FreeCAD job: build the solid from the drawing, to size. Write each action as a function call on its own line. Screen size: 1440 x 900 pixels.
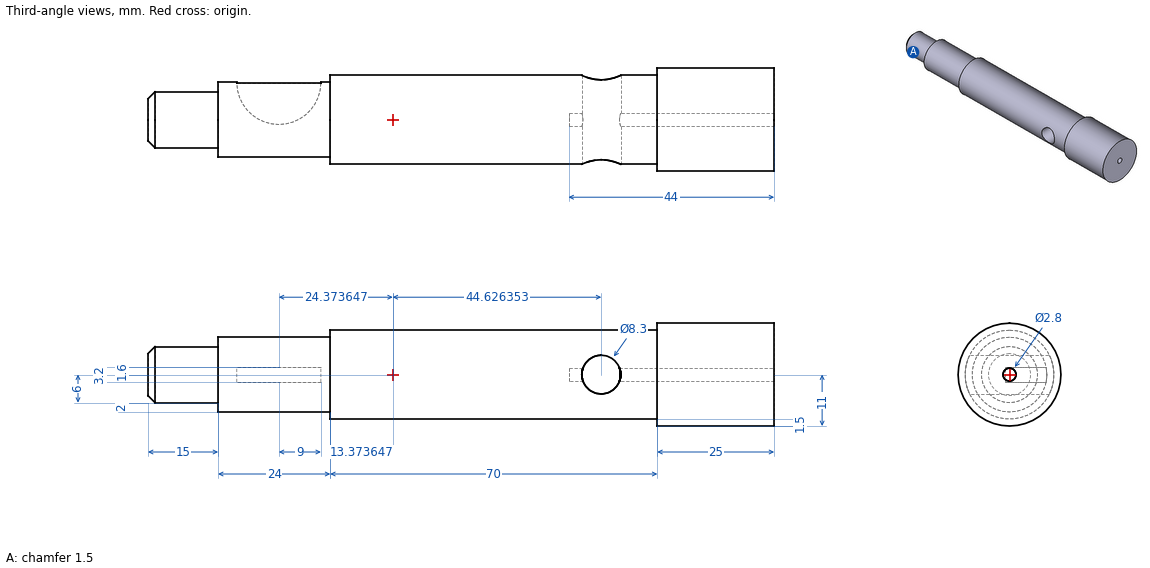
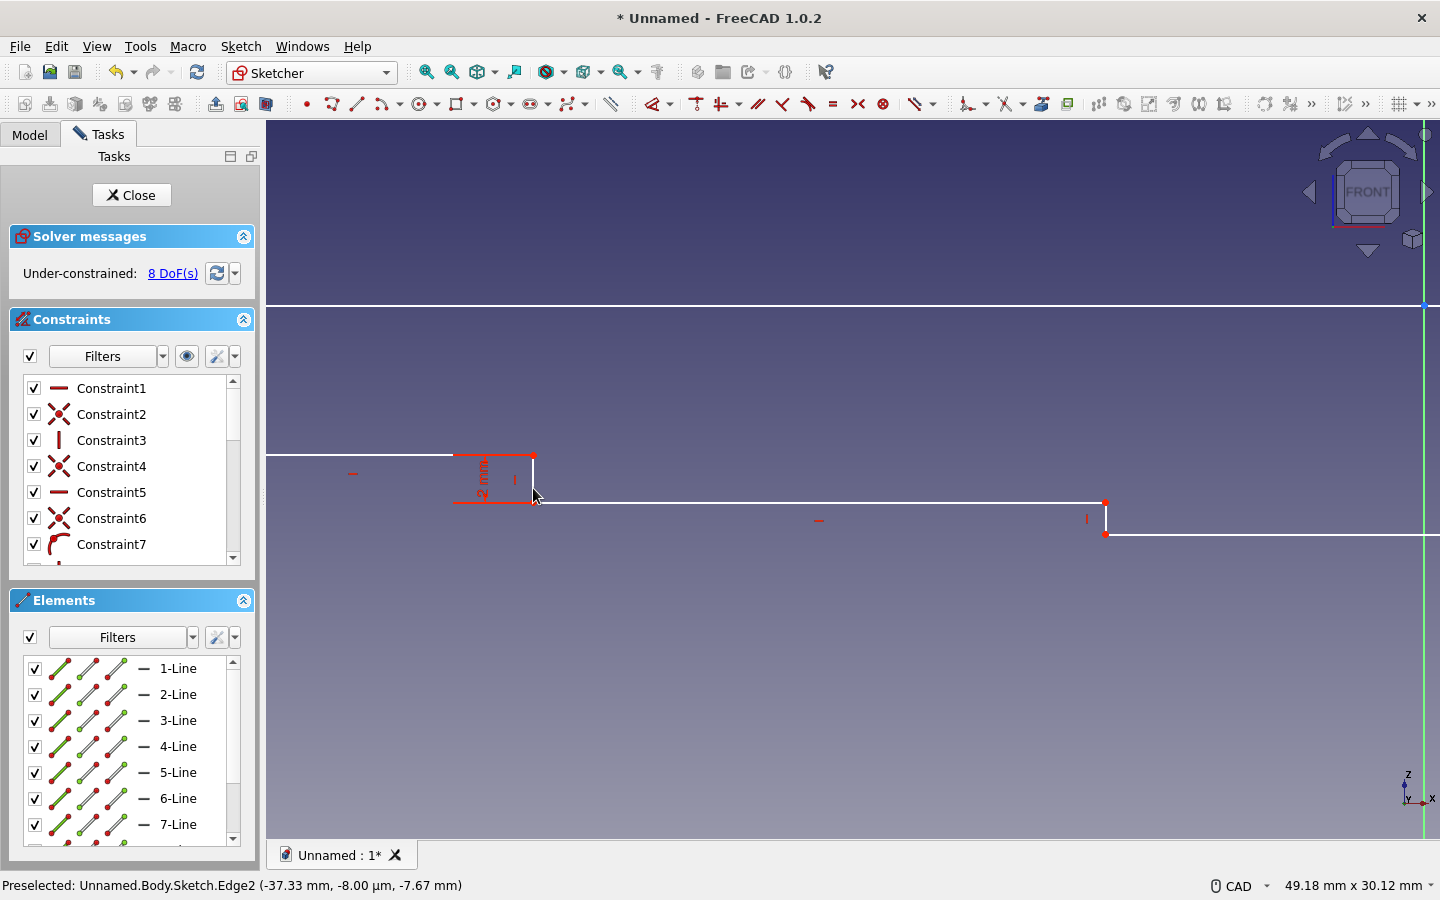
scroll(534, 490, down, 8)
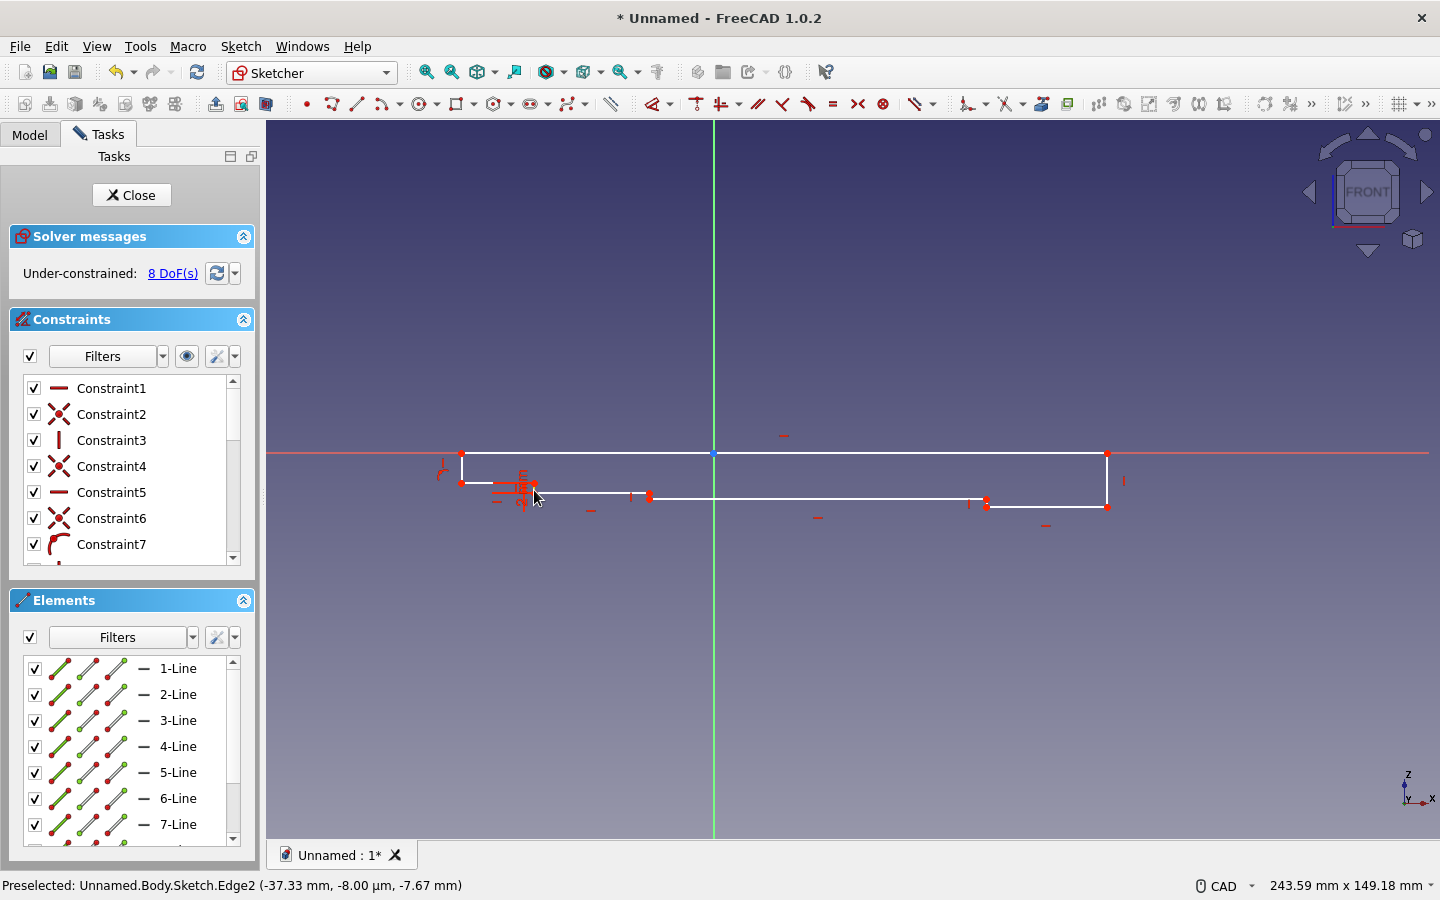
scroll(462, 474, up, 3)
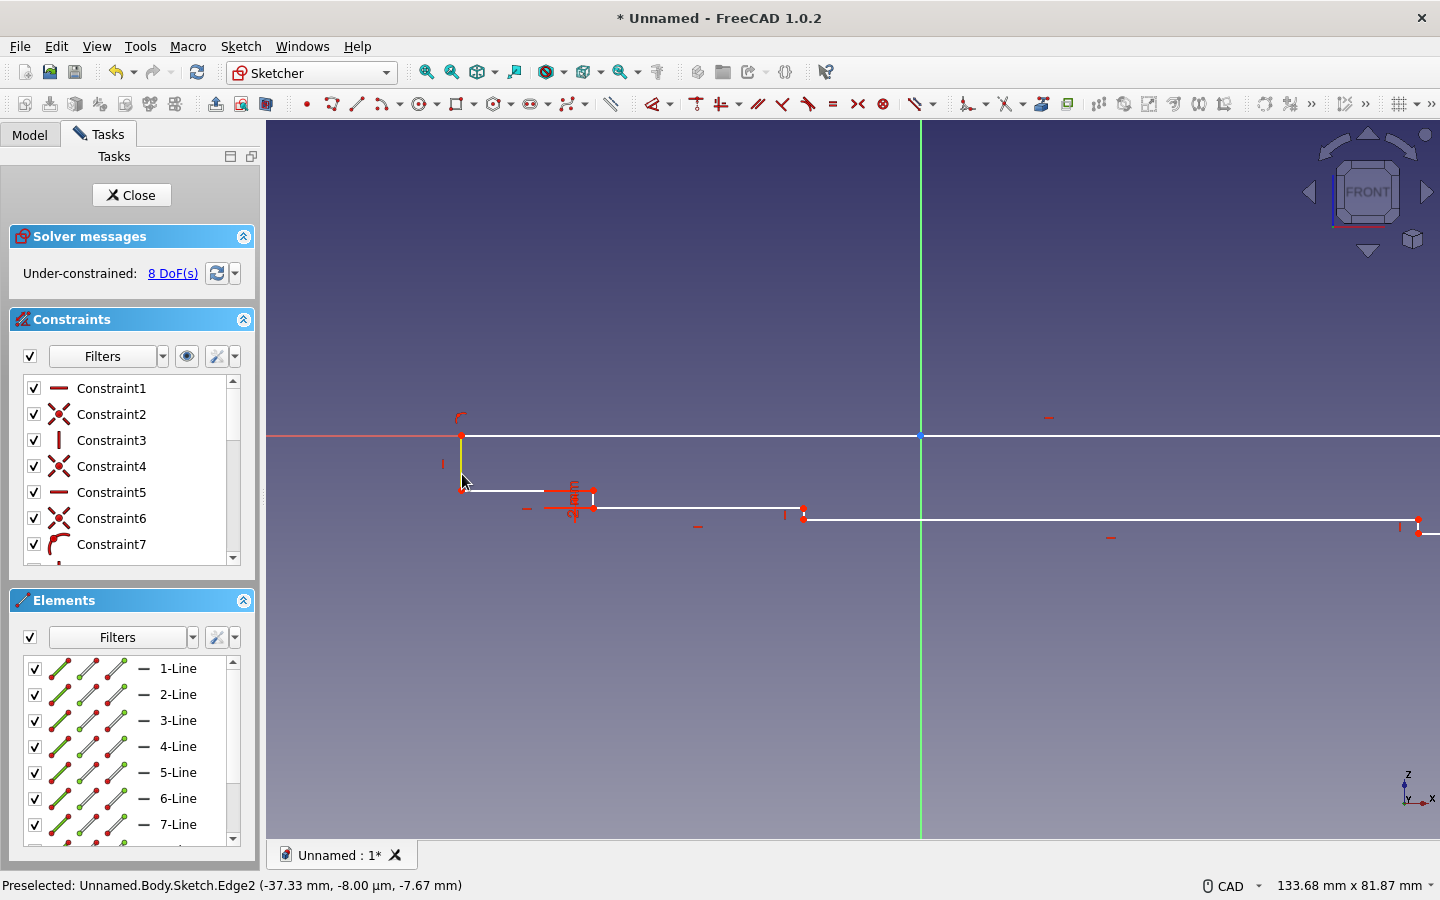
click(461, 474)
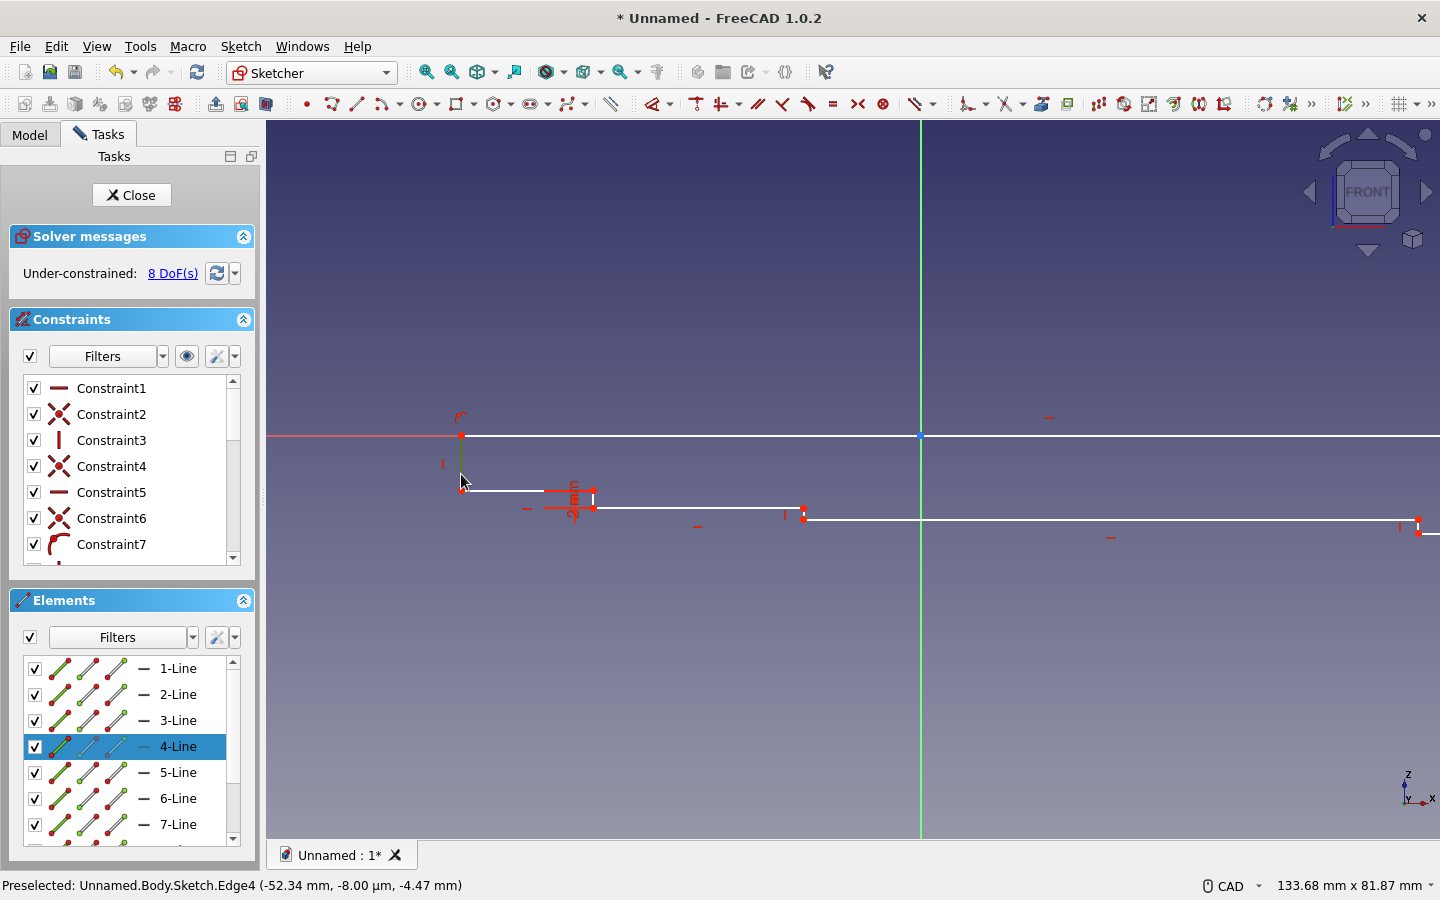
click(670, 104)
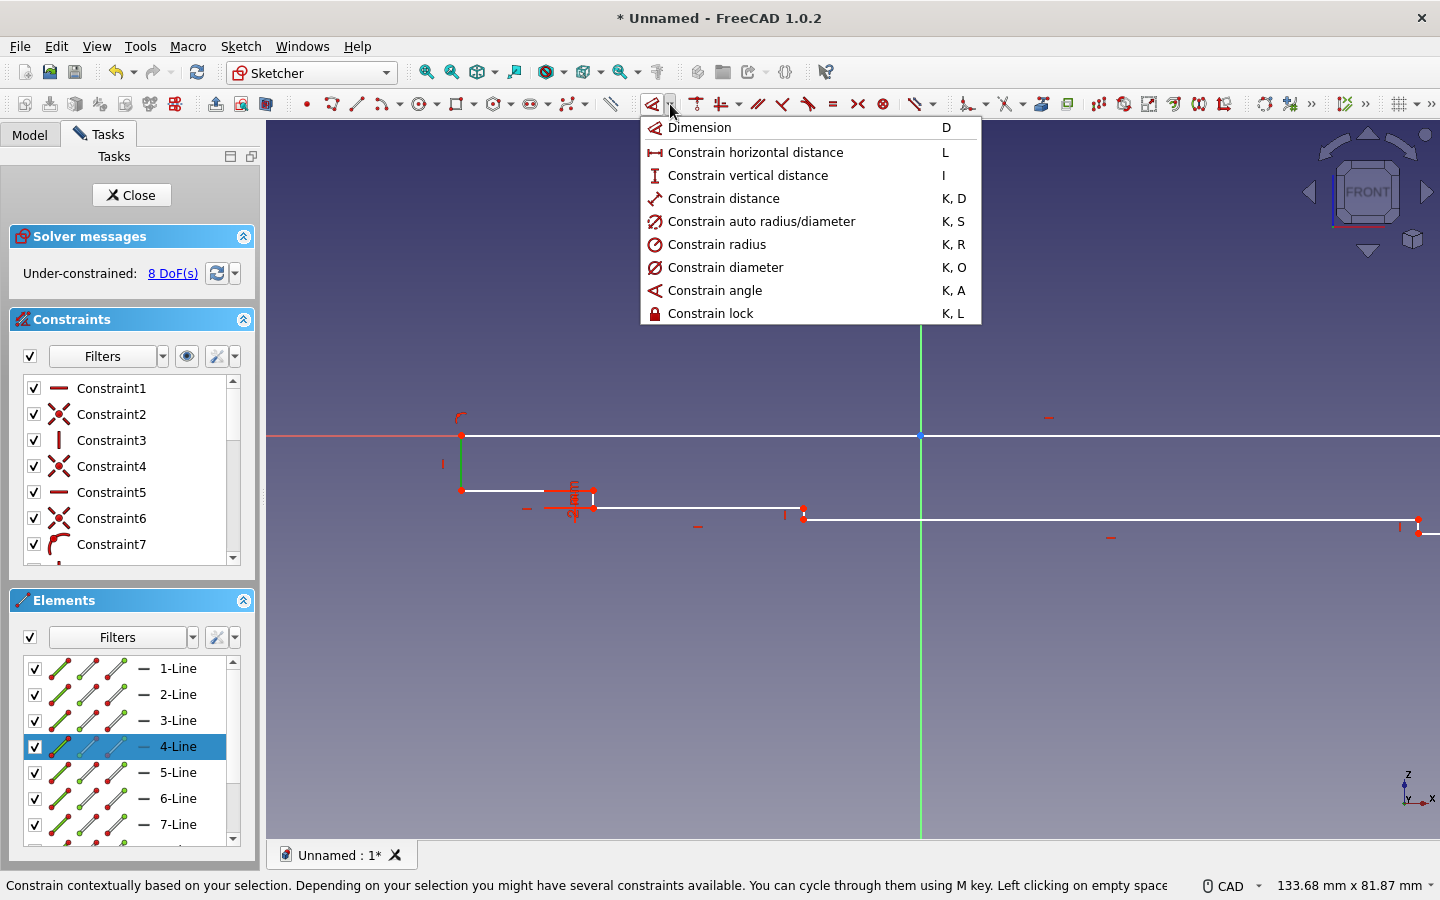
click(811, 176)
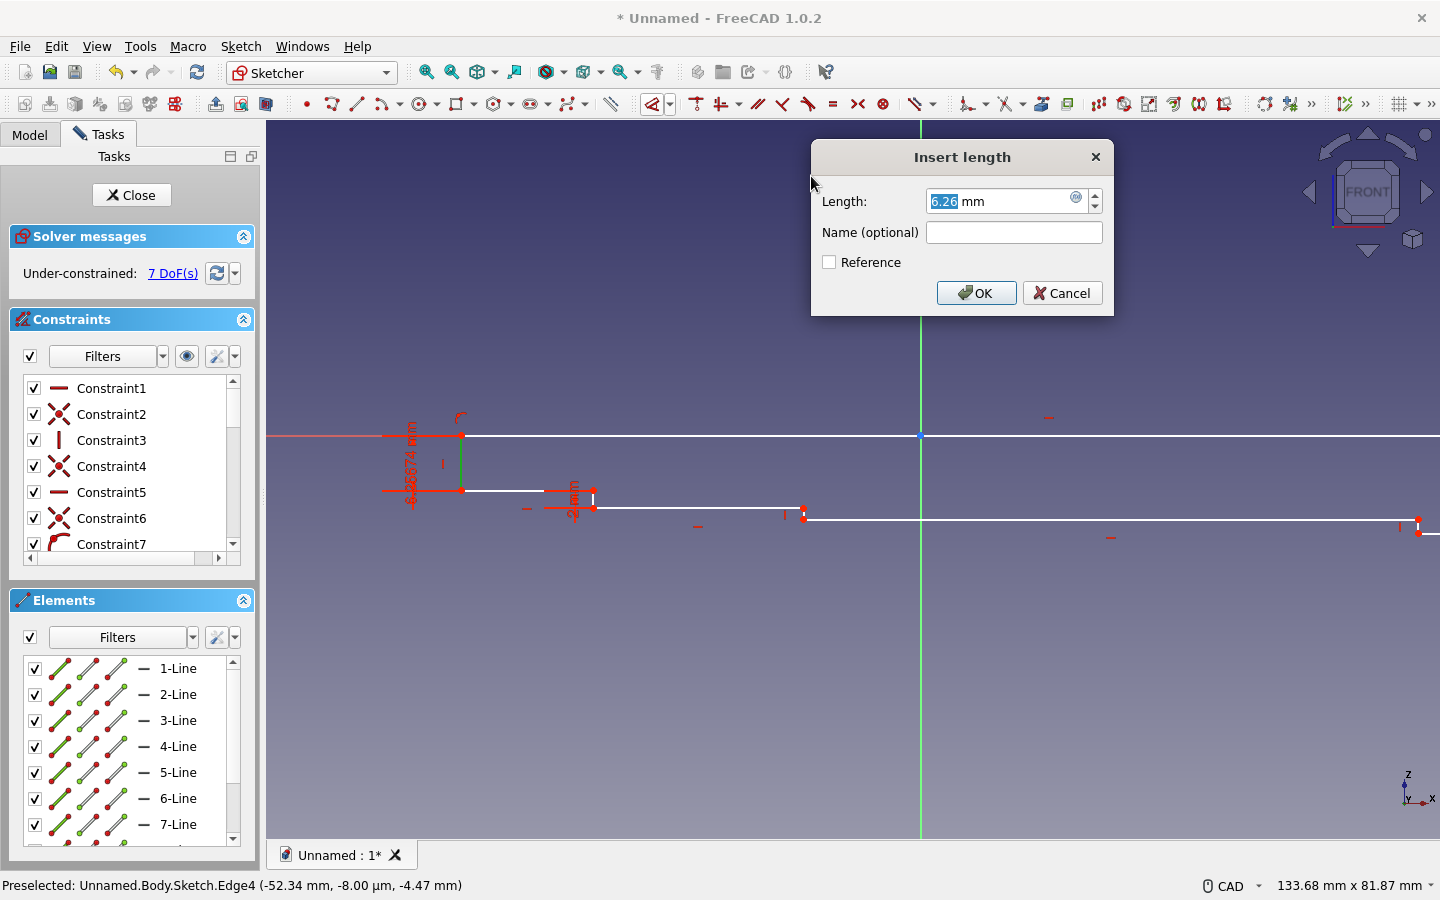
text(6)
key(Return)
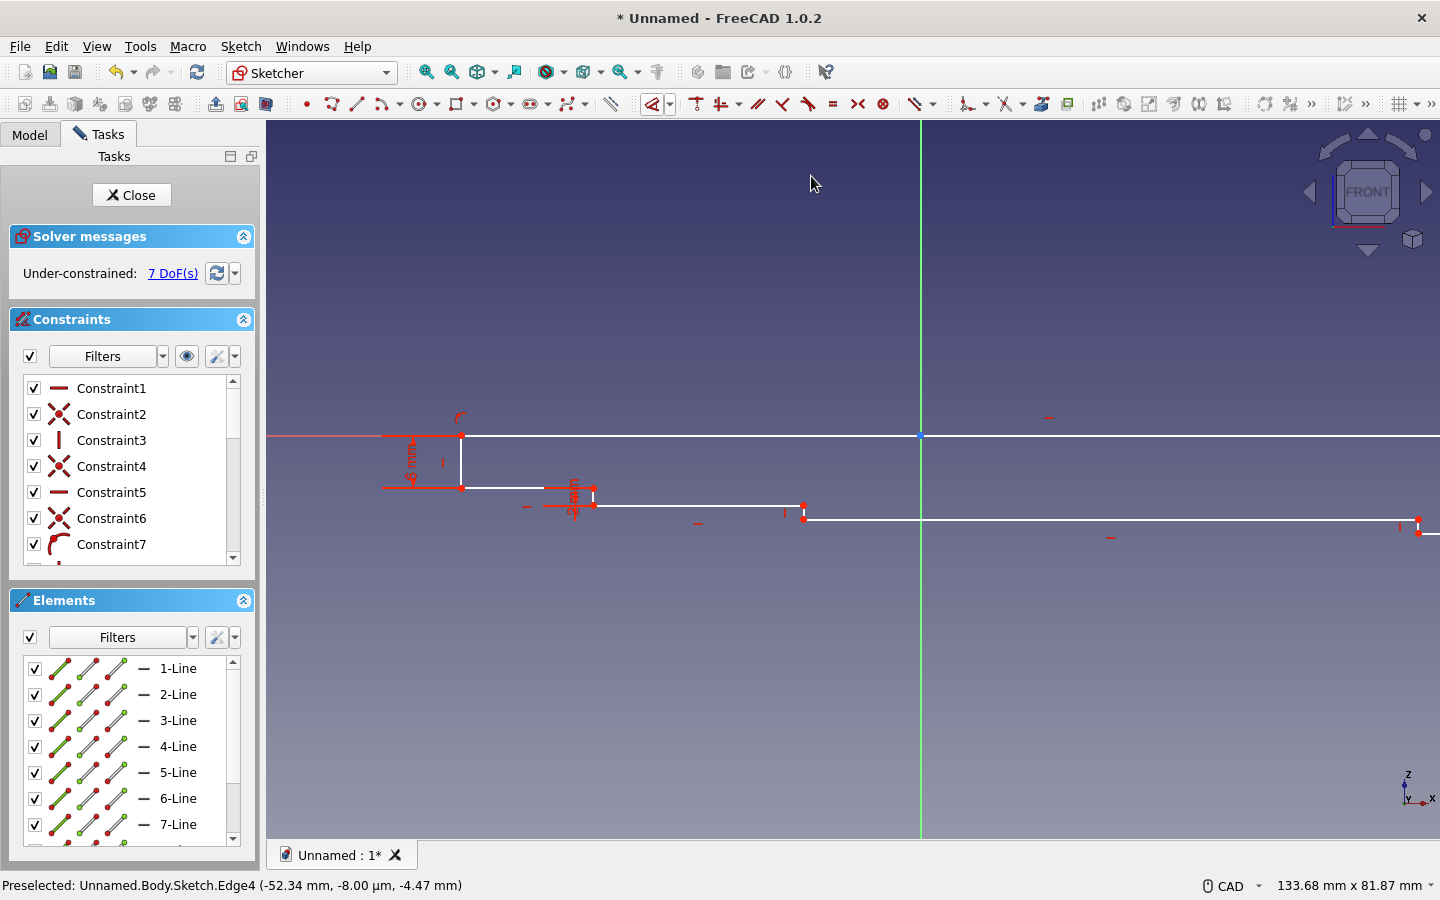
click(741, 506)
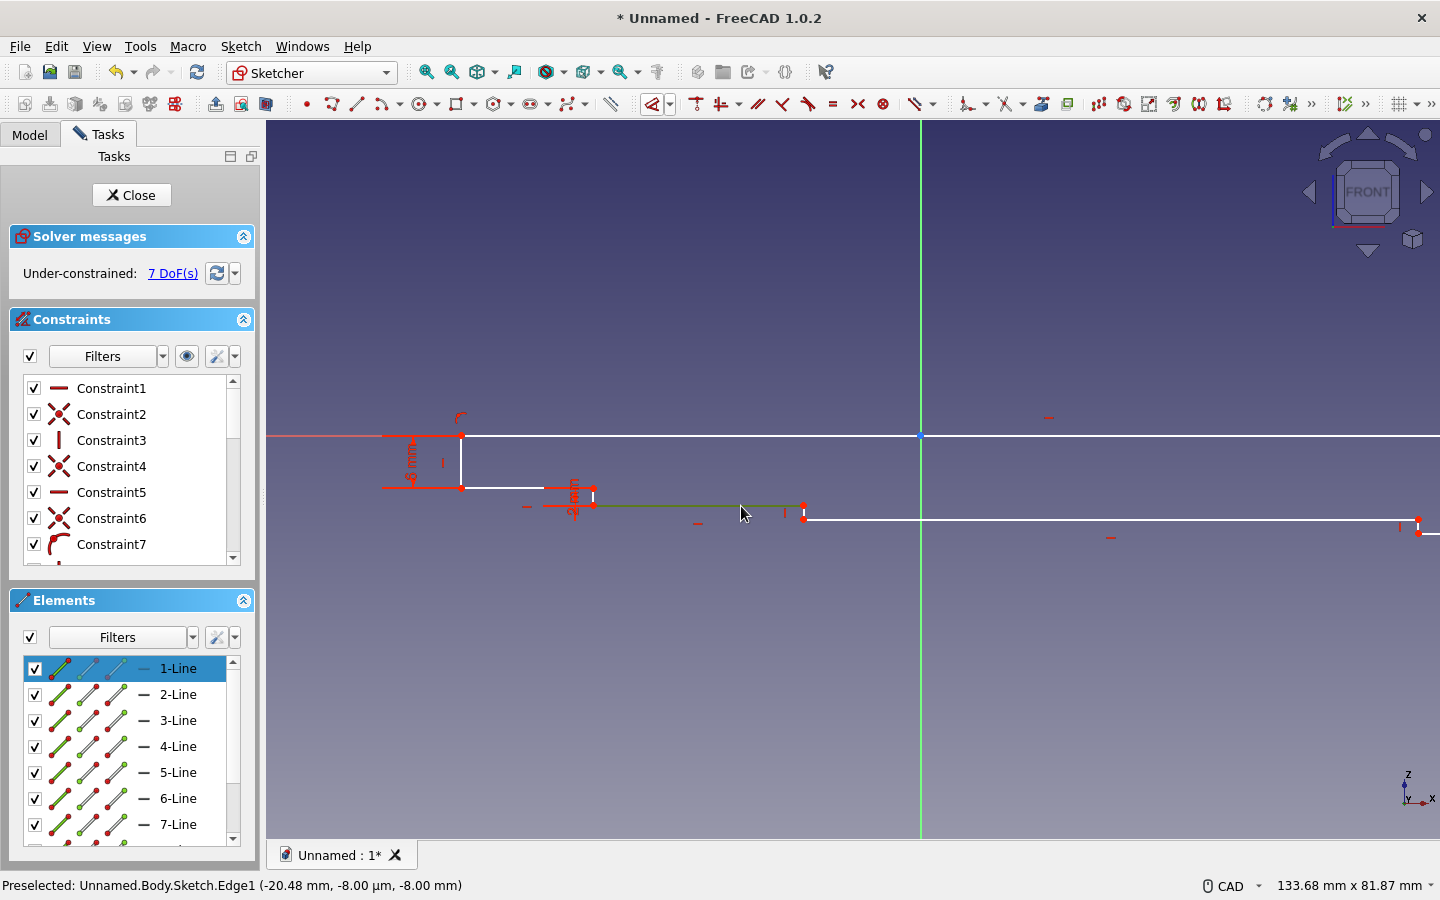
key(l)